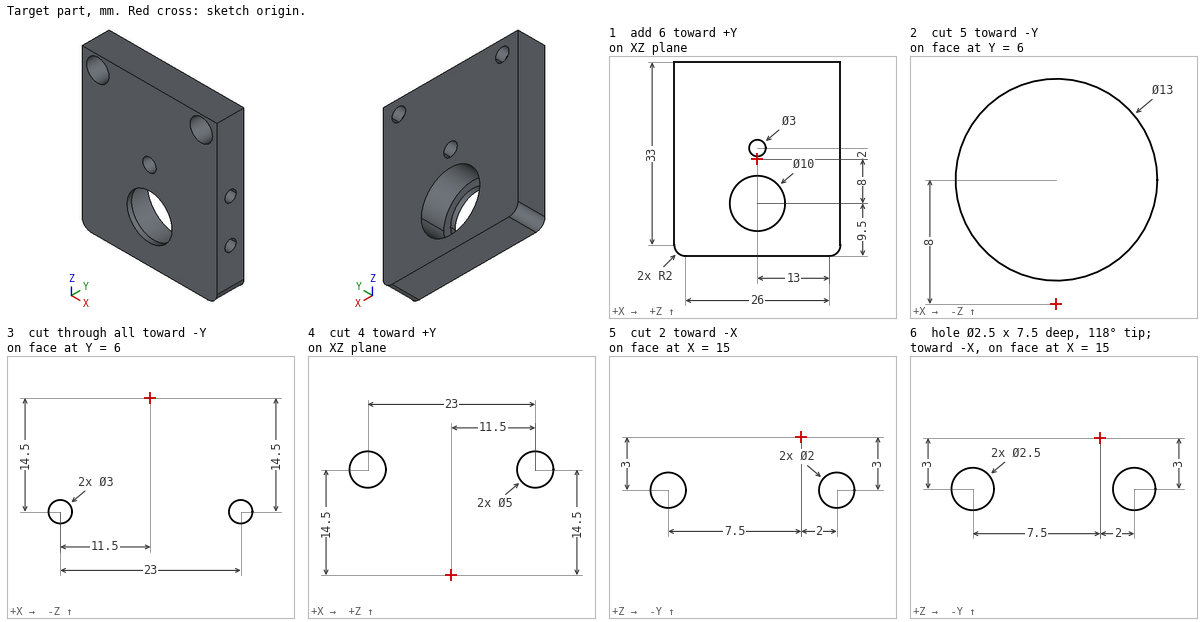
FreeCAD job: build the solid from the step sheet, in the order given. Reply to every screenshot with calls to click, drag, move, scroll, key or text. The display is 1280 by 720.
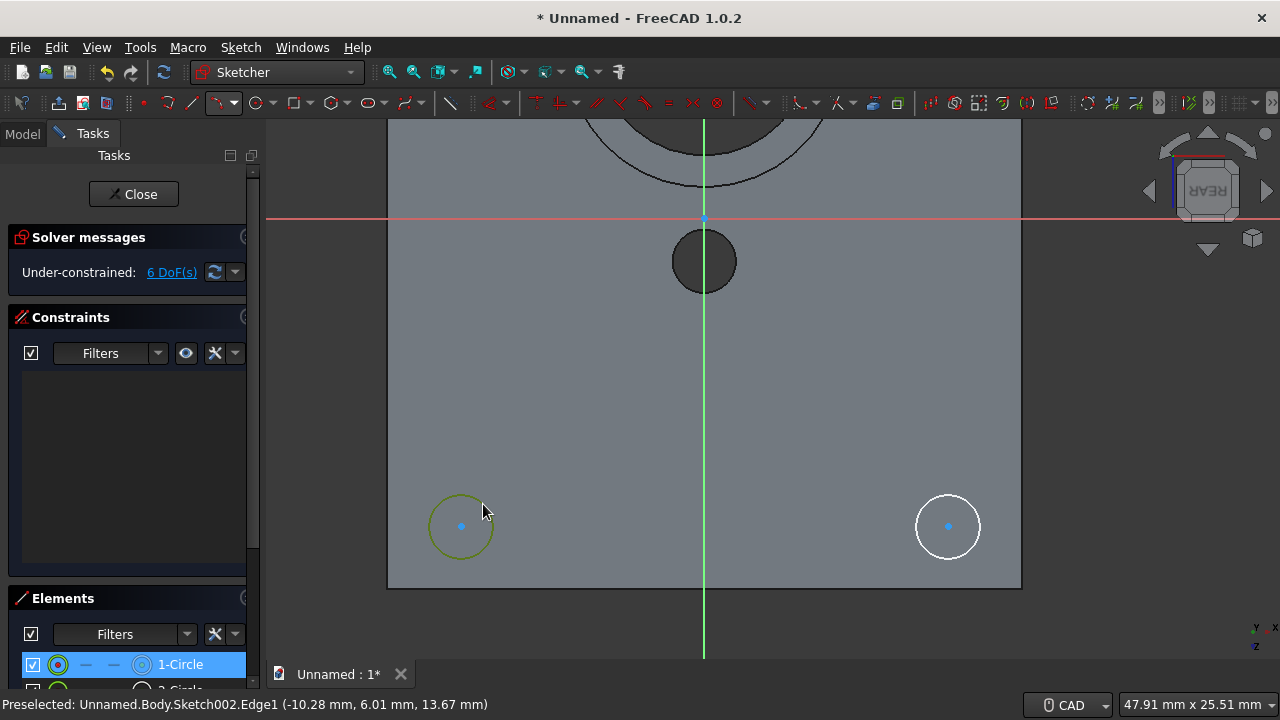
click(970, 504)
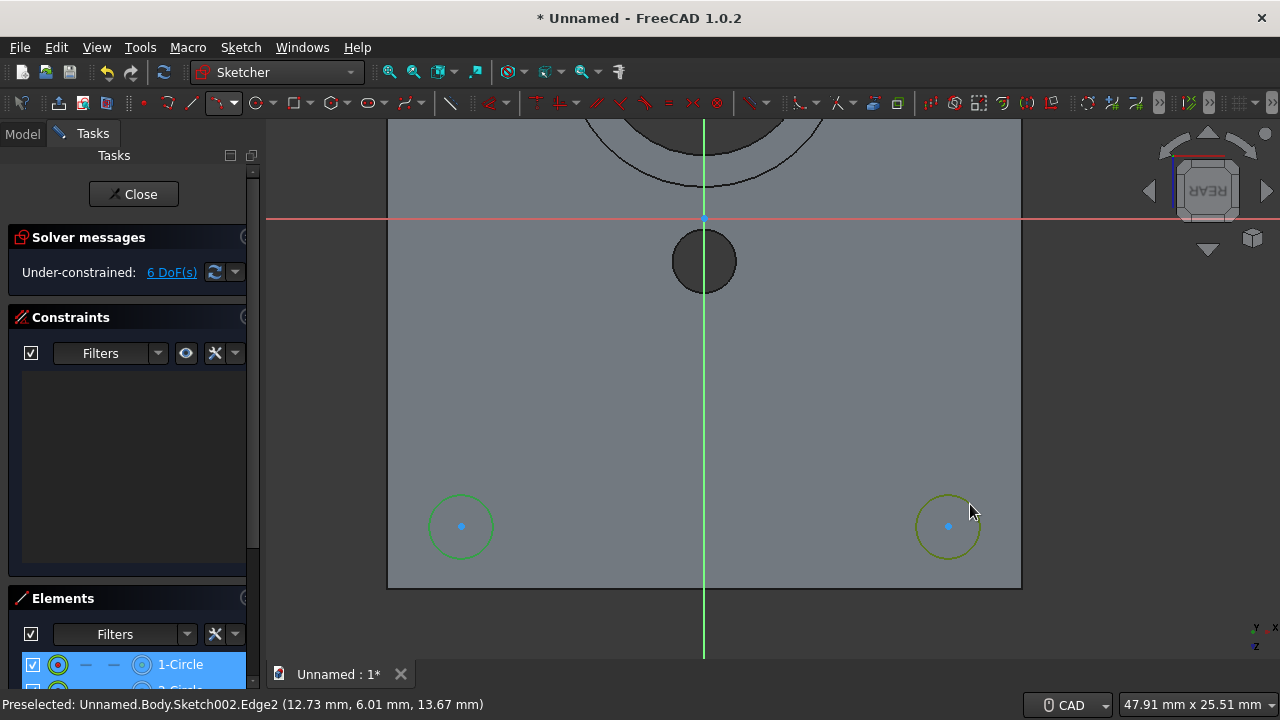
key(e)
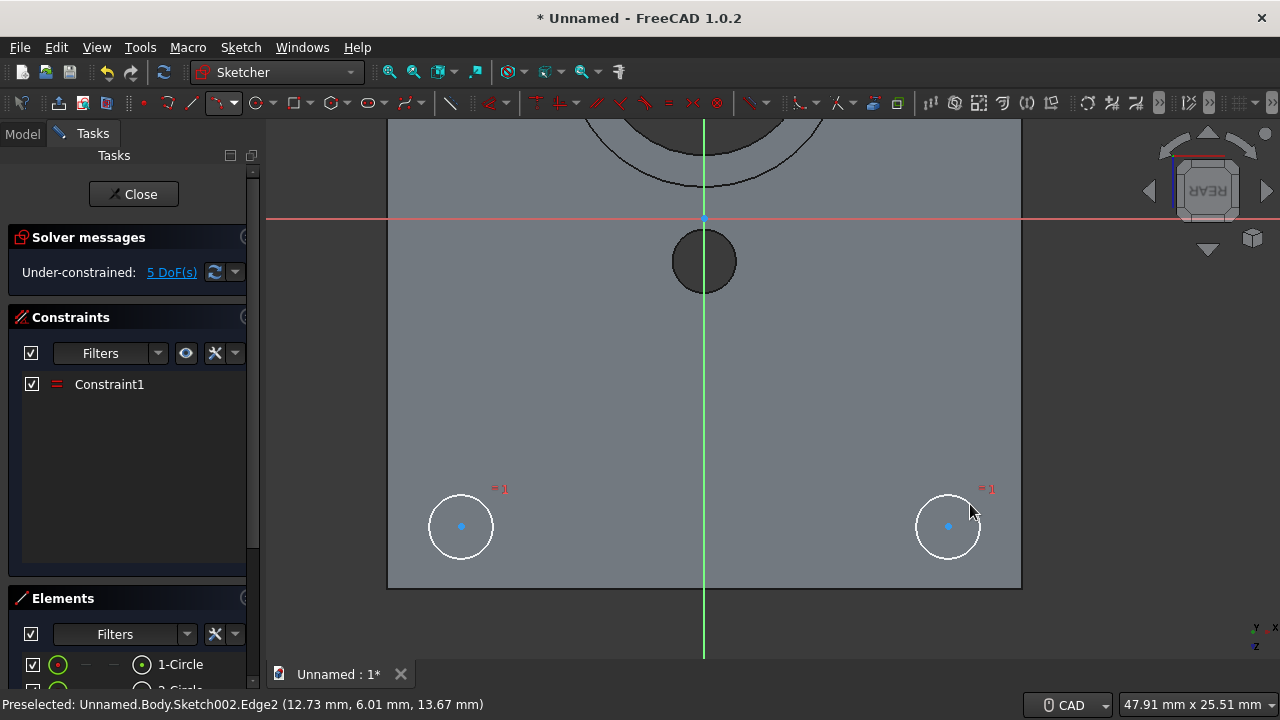
click(490, 104)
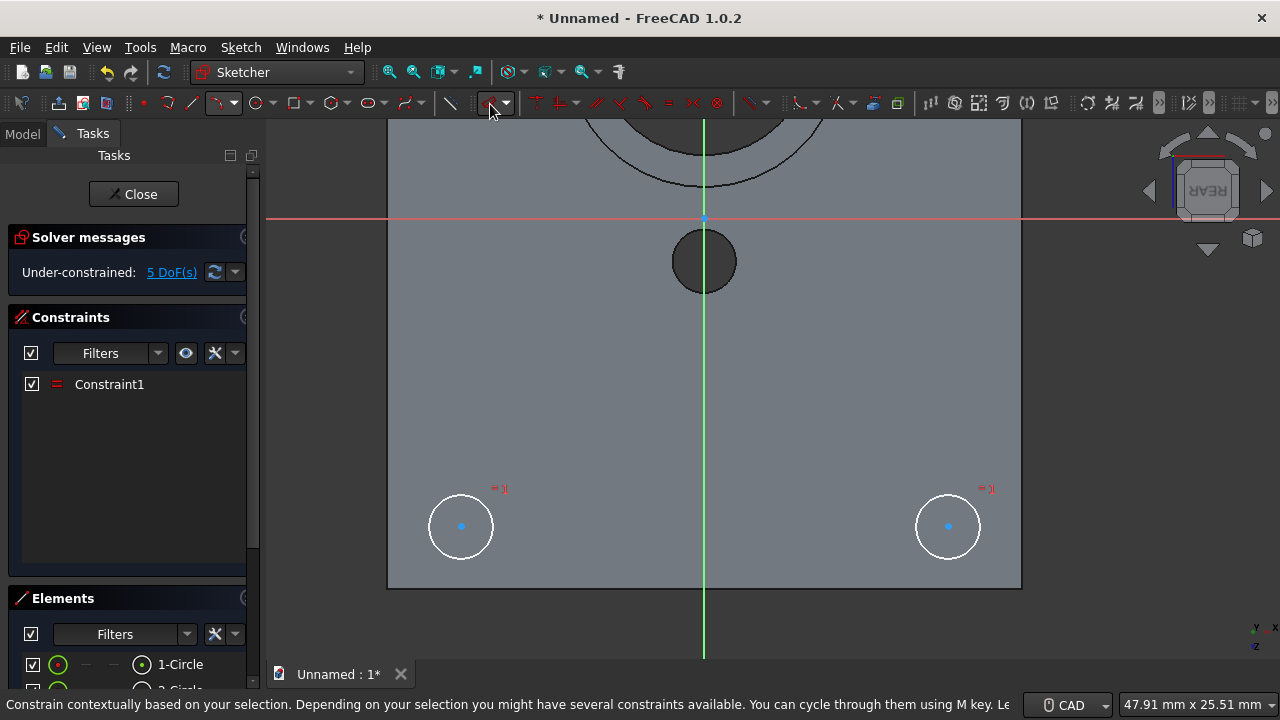
click(483, 504)
click(505, 481)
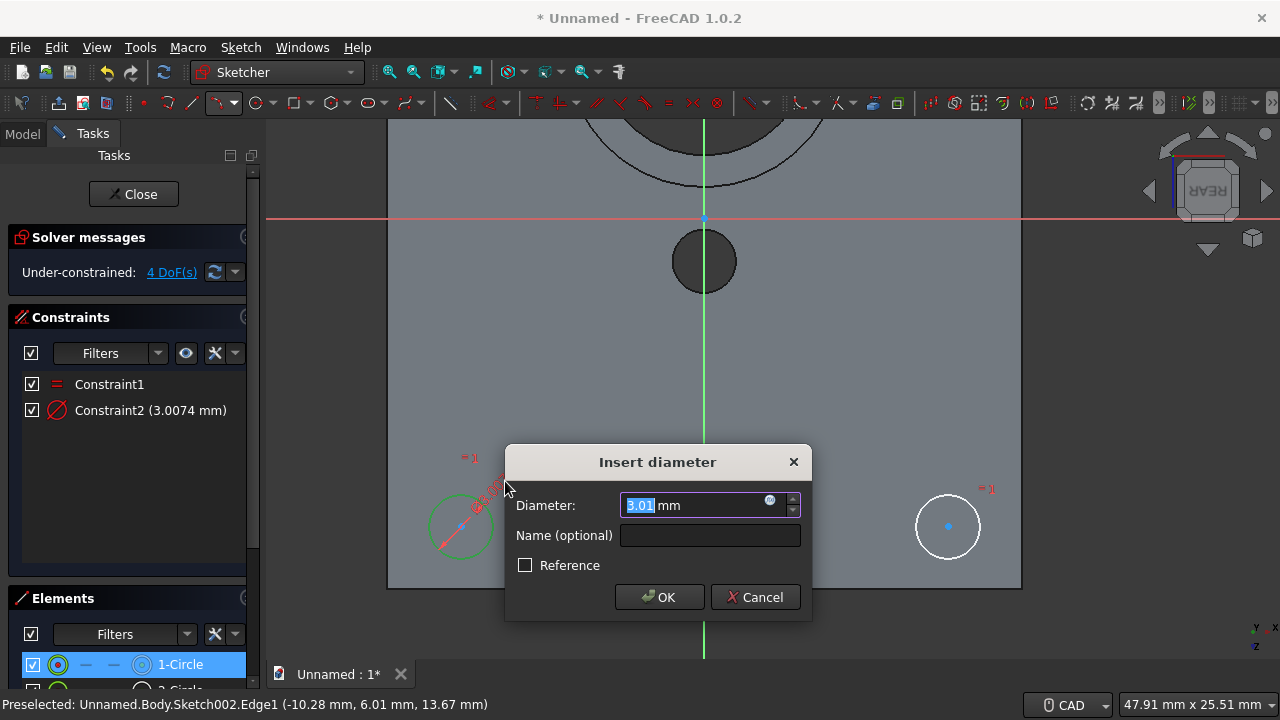
text(3)
key(Return)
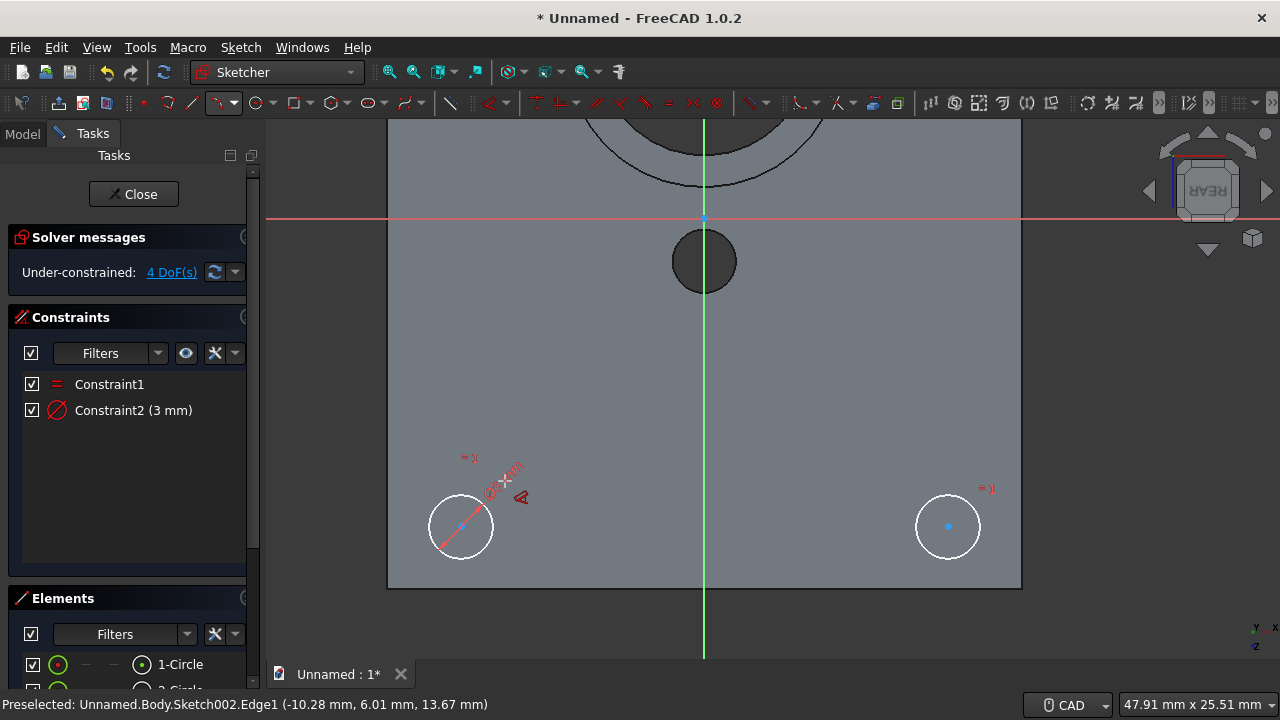
click(461, 527)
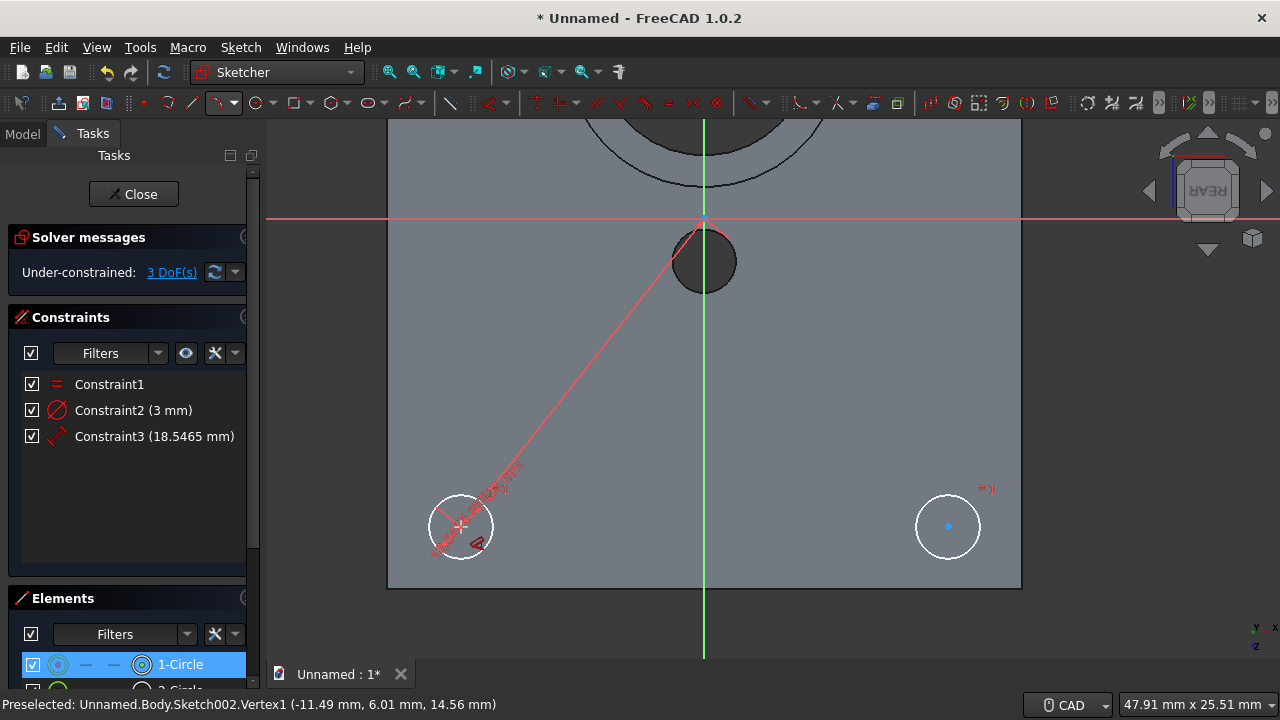
click(948, 527)
click(592, 561)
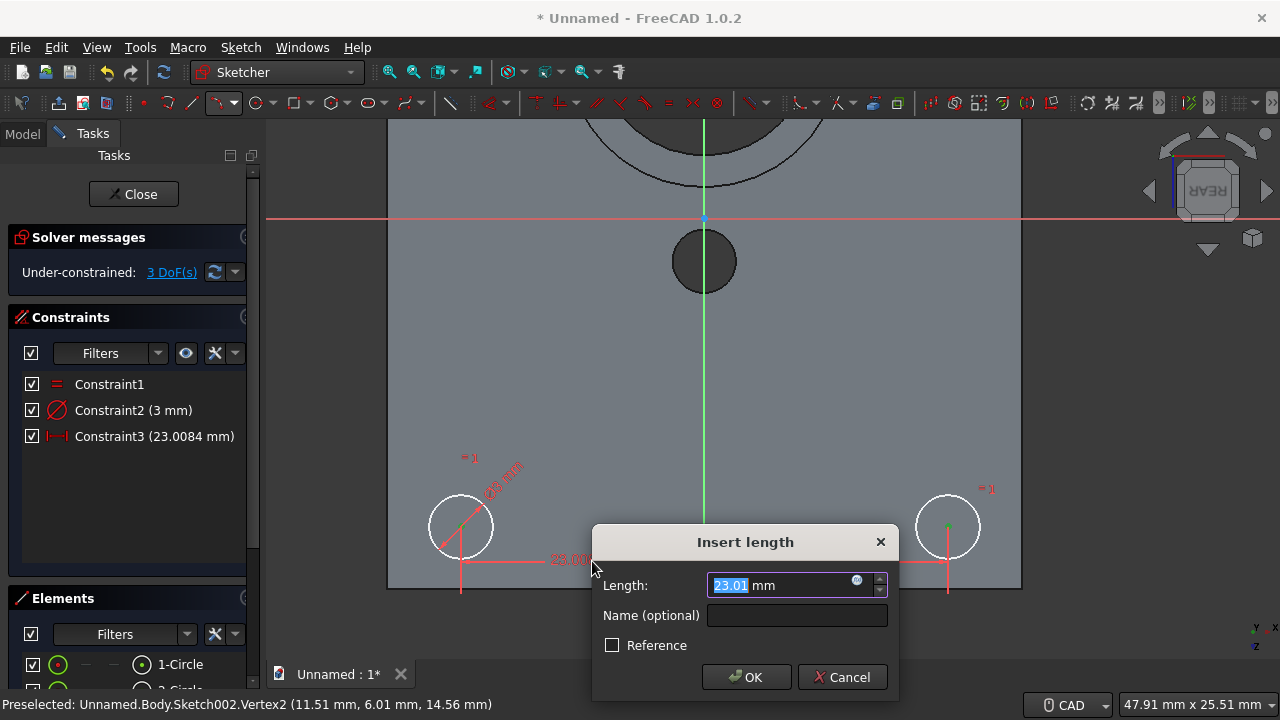
text(23)
key(Return)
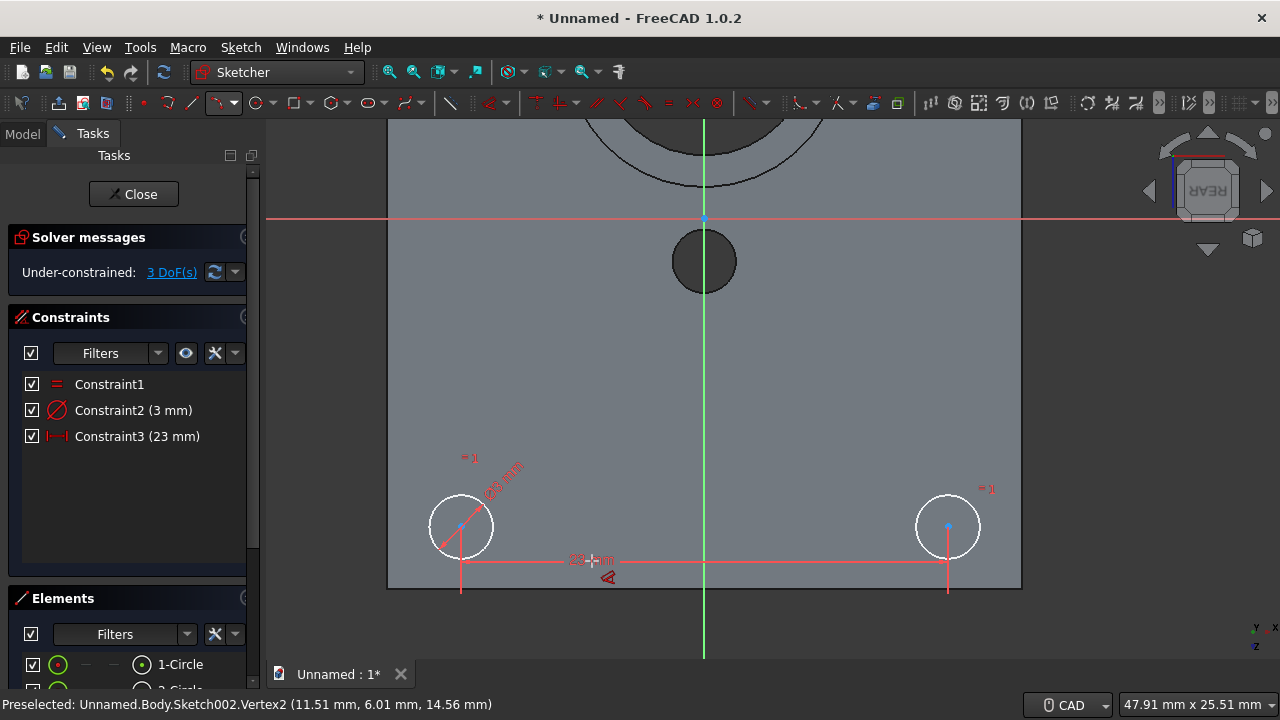
click(461, 527)
click(583, 185)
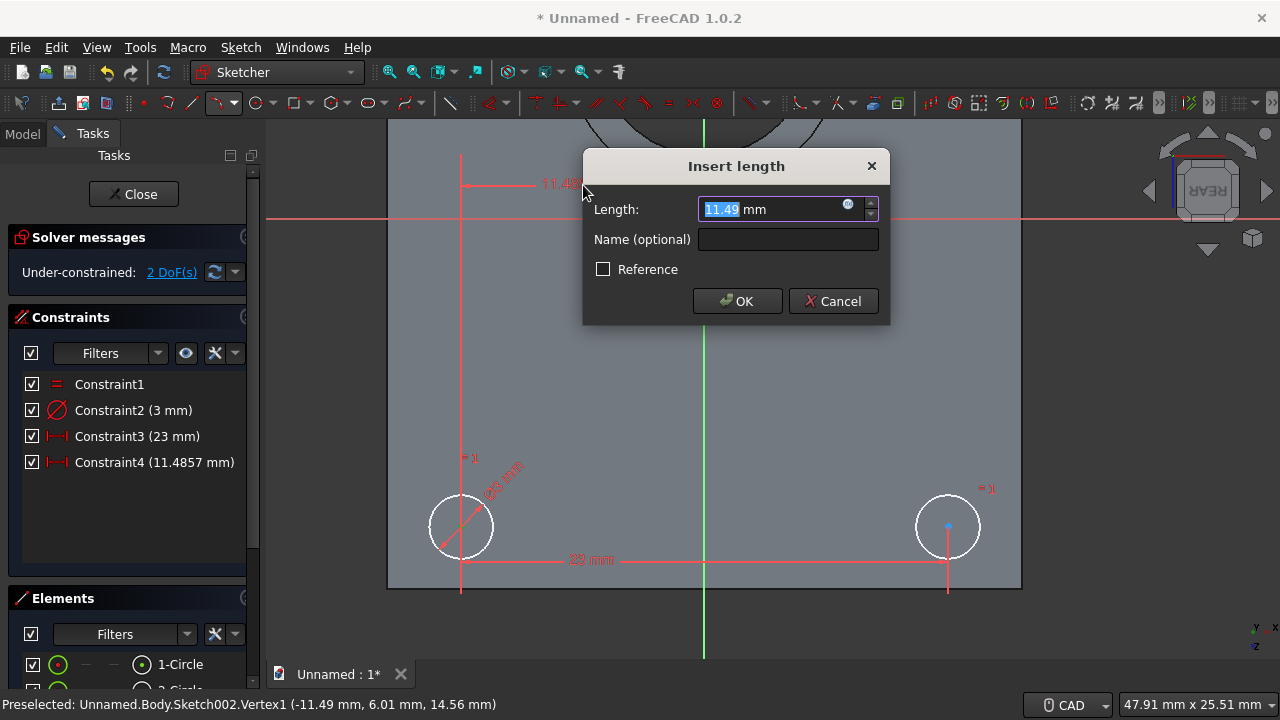
text(11.5)
key(Return)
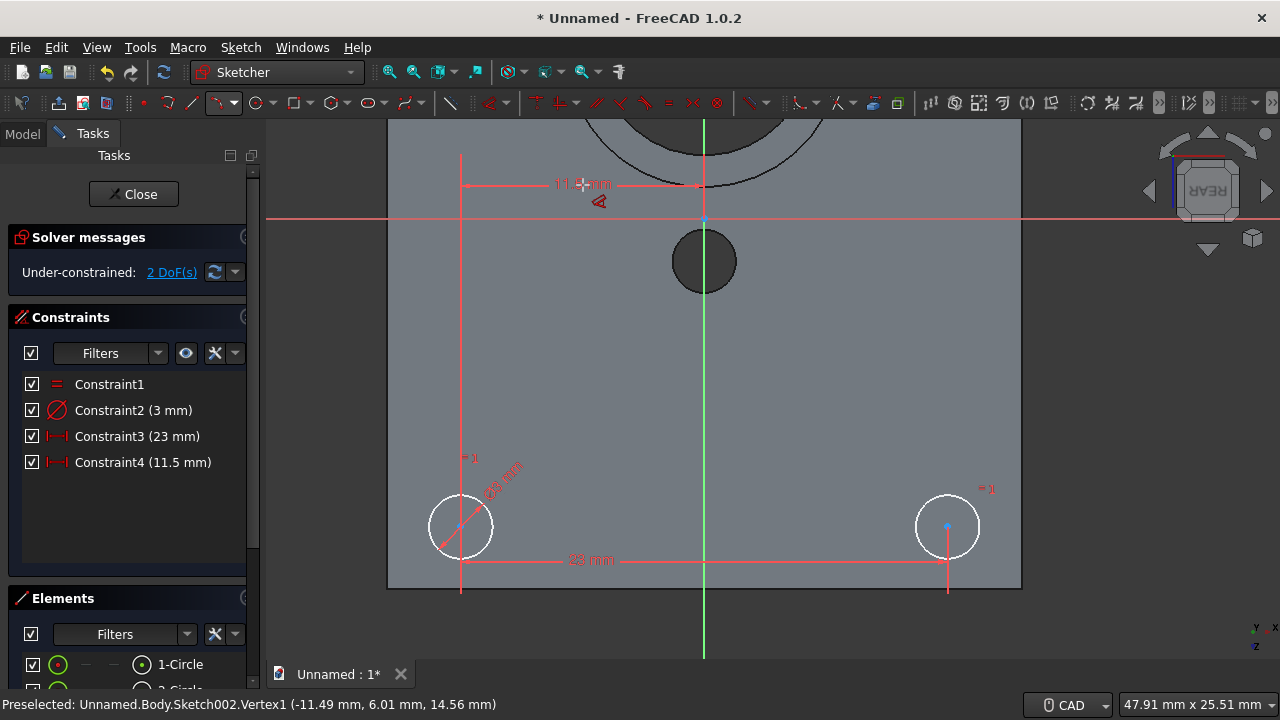
click(461, 527)
click(427, 373)